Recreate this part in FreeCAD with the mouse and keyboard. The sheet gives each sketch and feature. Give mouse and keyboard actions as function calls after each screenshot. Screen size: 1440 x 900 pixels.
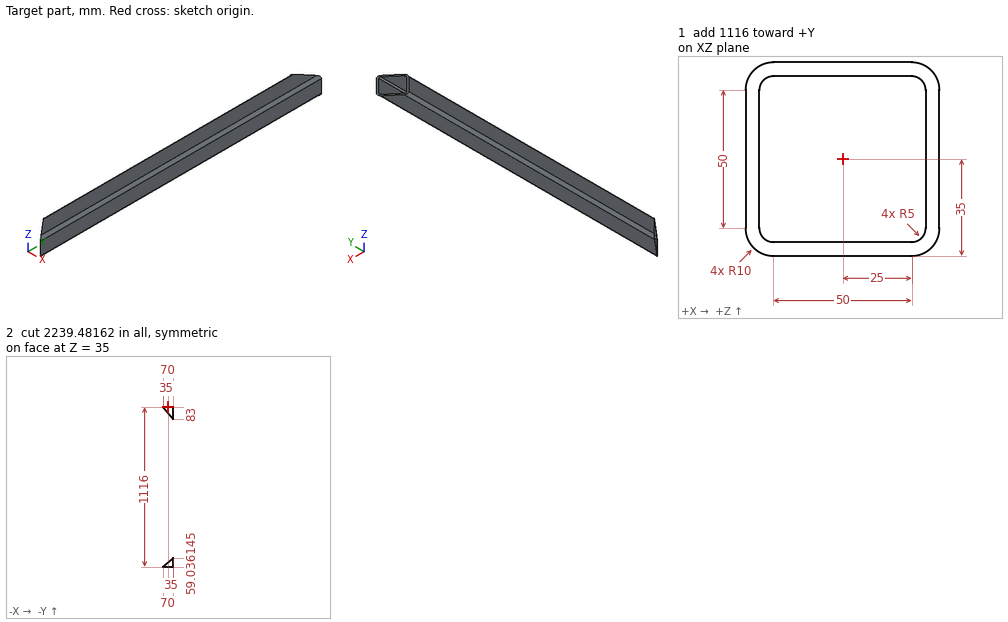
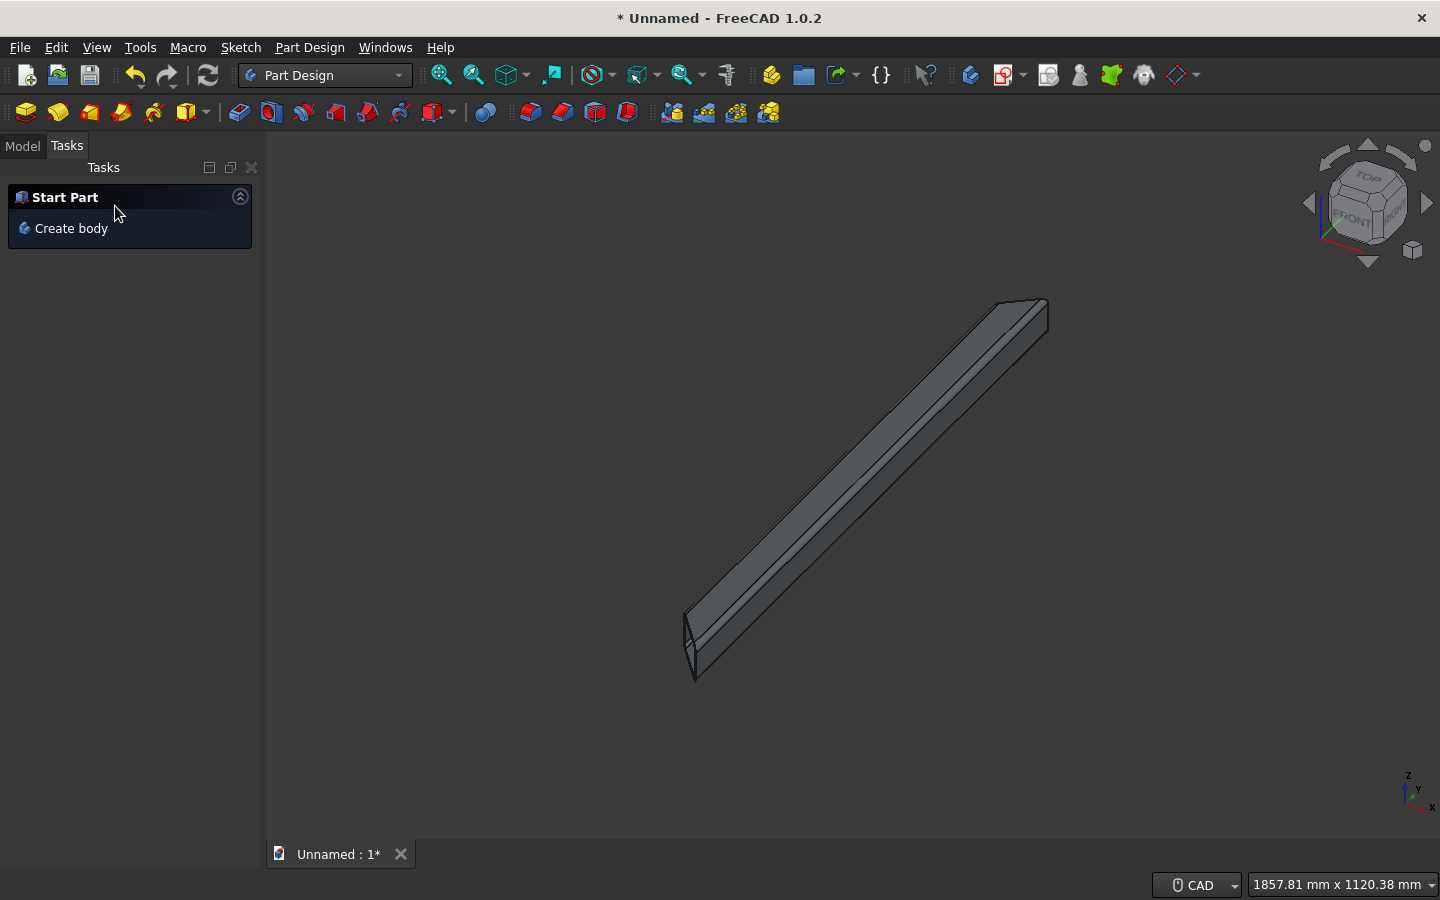
key(0)